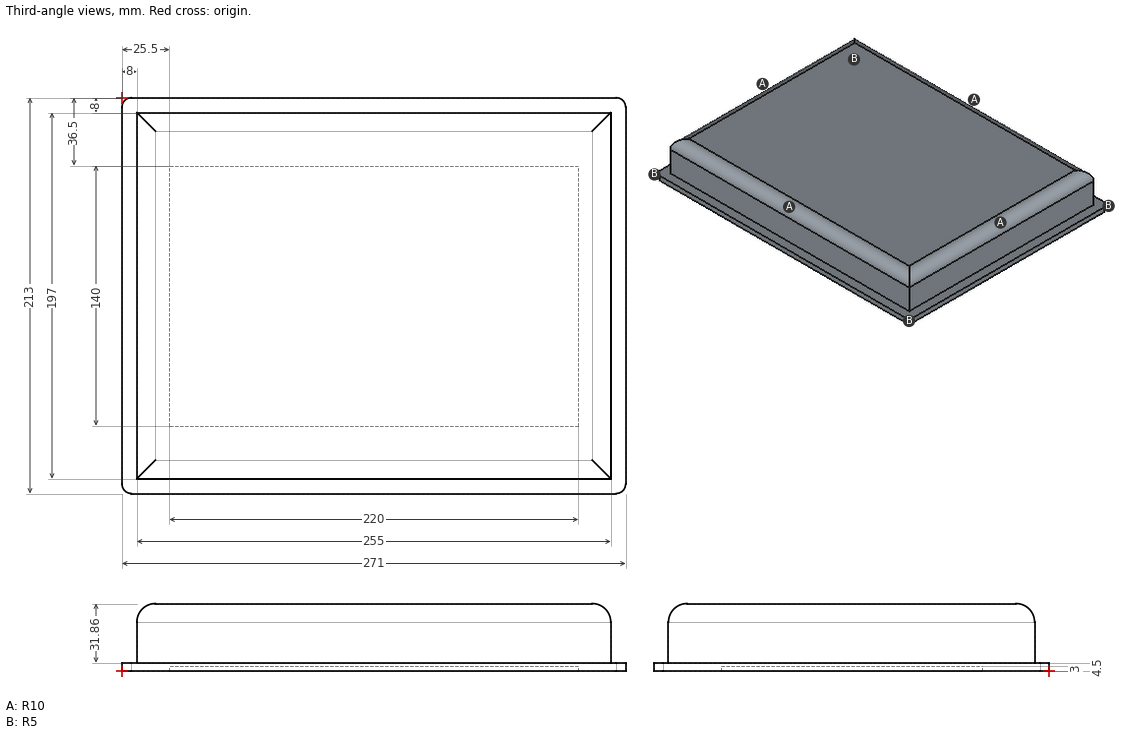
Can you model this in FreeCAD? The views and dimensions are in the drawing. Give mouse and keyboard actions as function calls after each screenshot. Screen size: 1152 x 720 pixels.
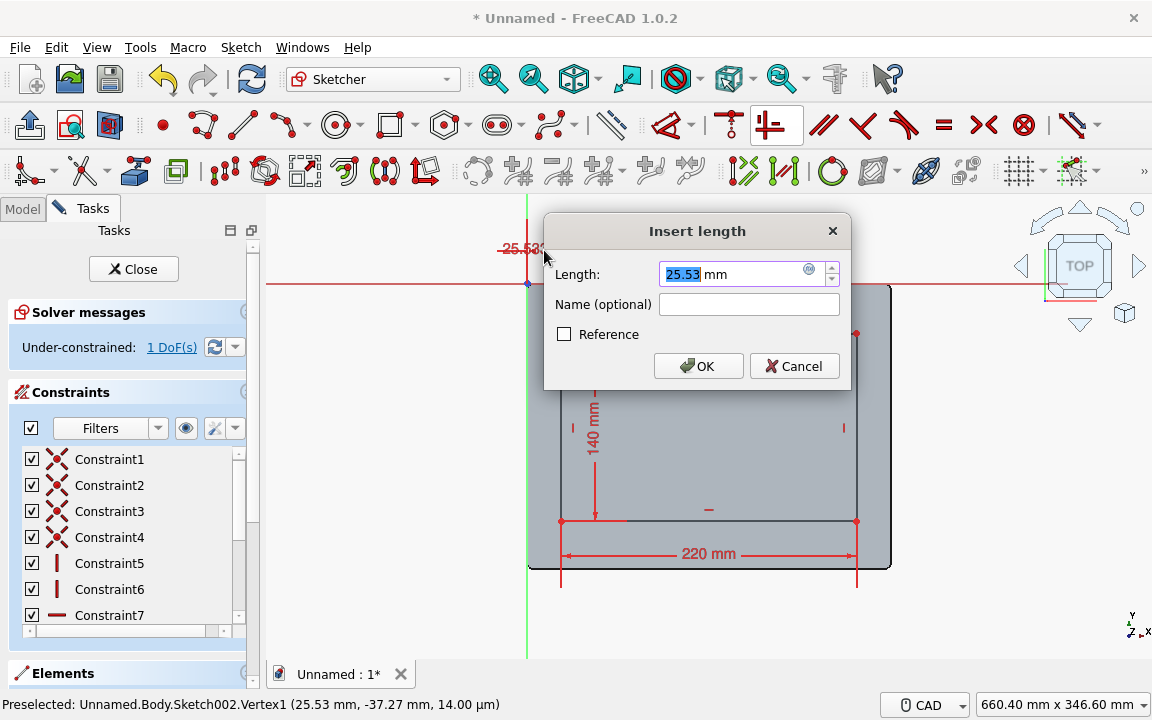
text(25.5)
key(Return)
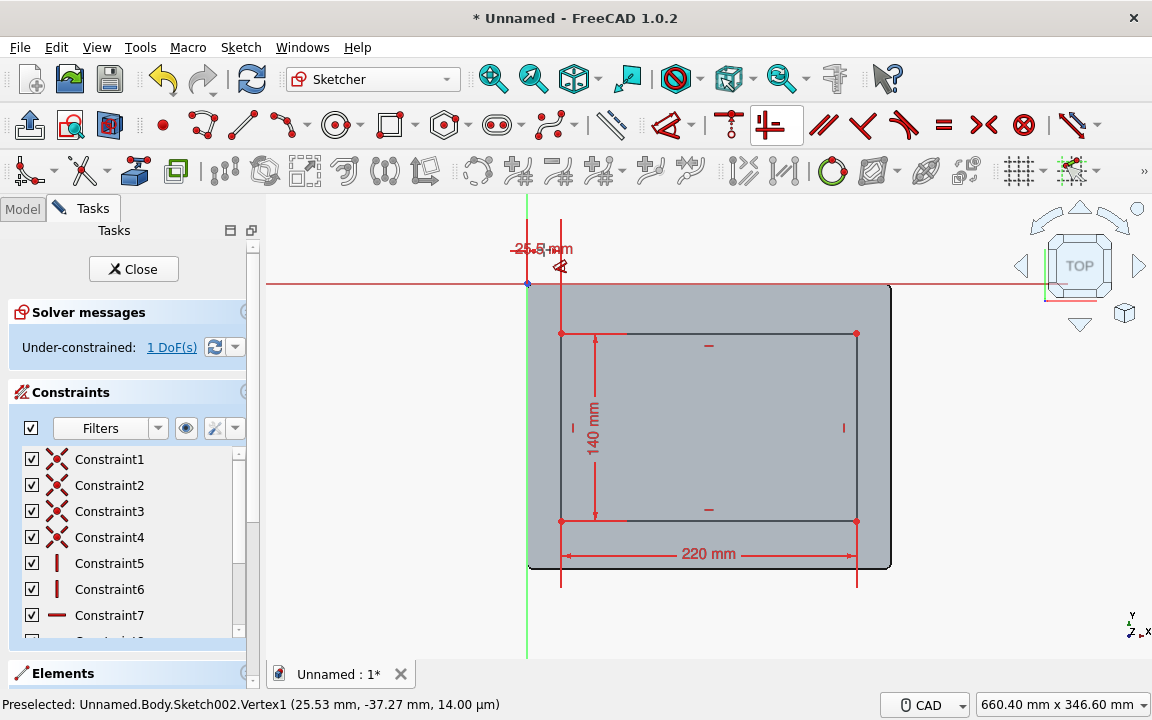
click(561, 334)
click(493, 309)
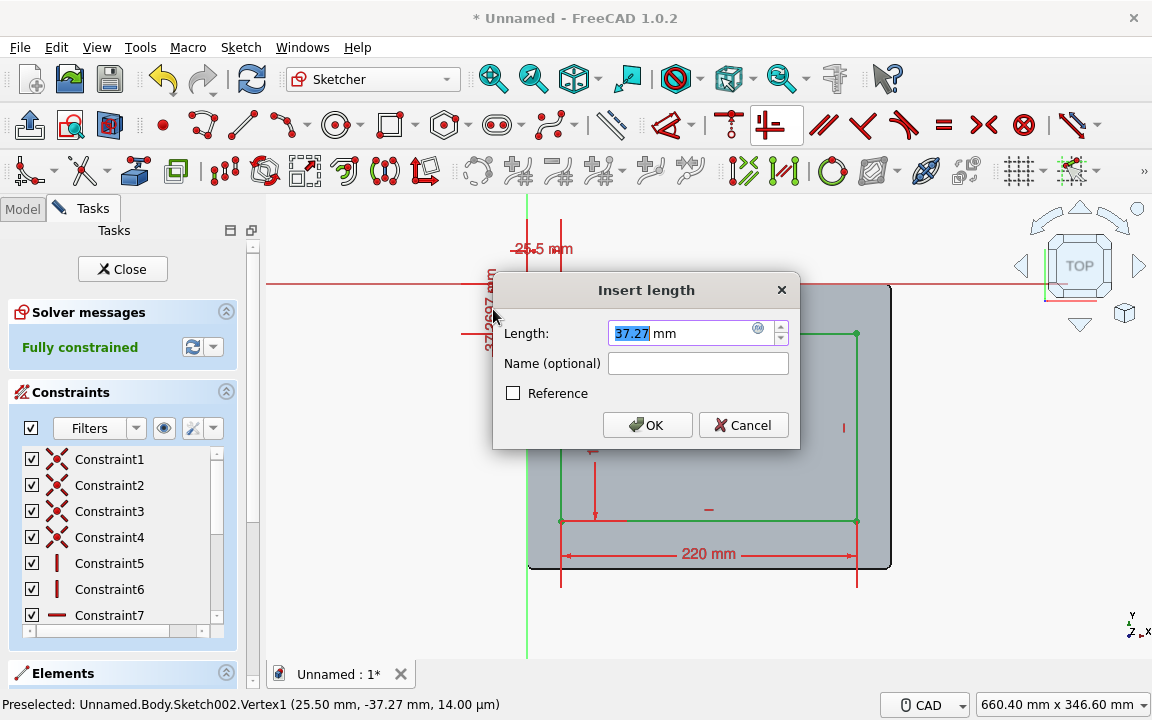
text(36.5)
key(Return)
key(Escape)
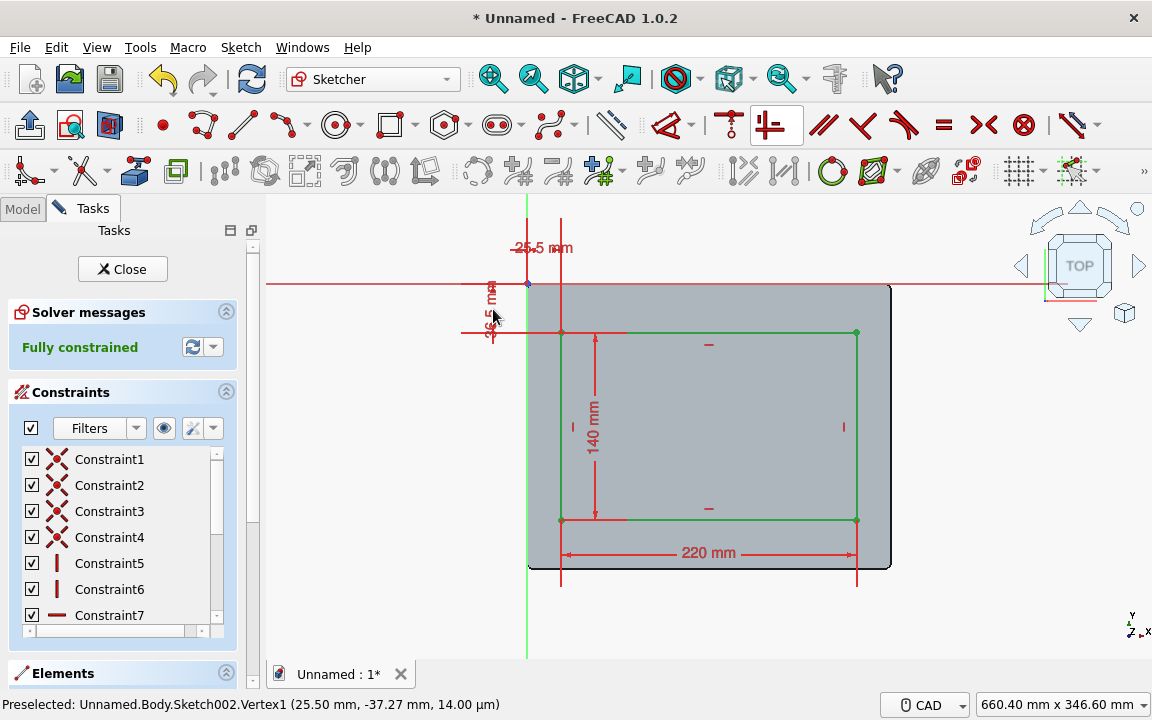
click(123, 269)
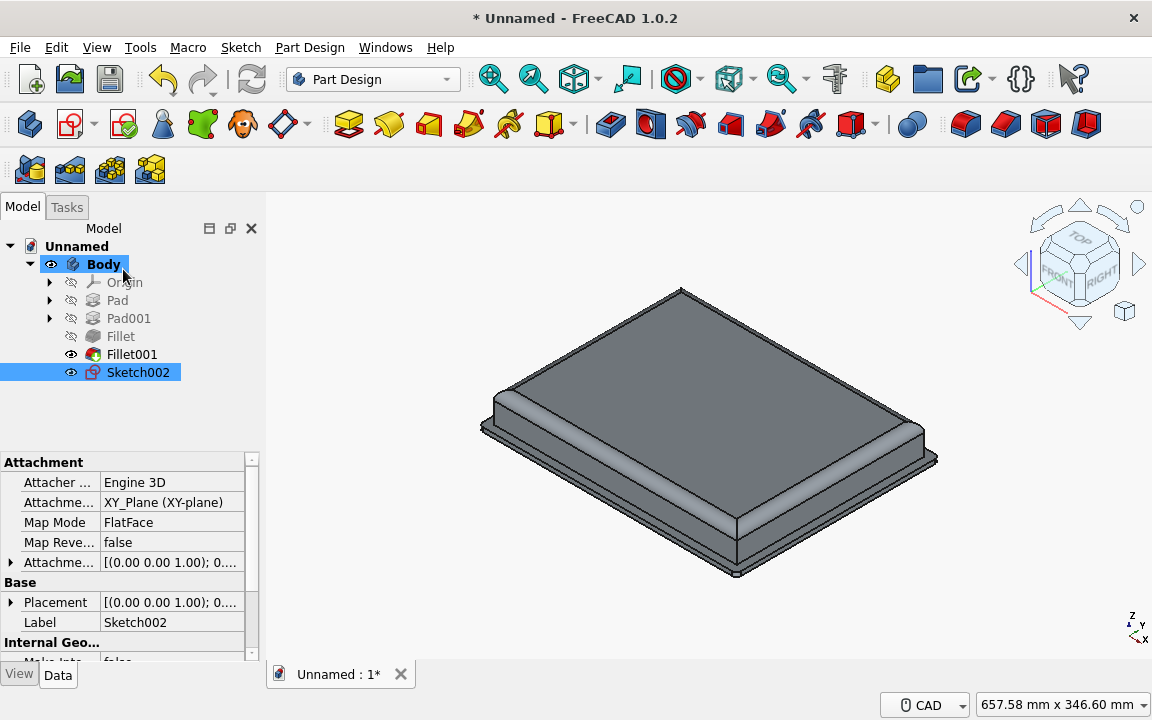
click(612, 124)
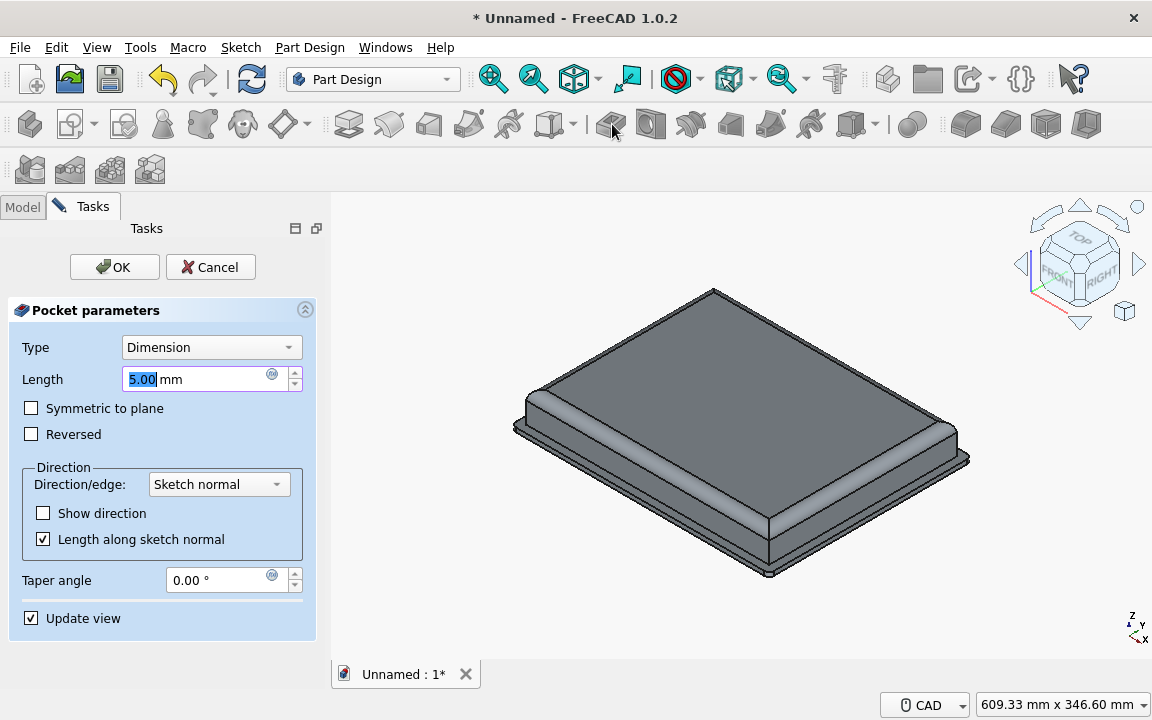
text(3)
key(Tab)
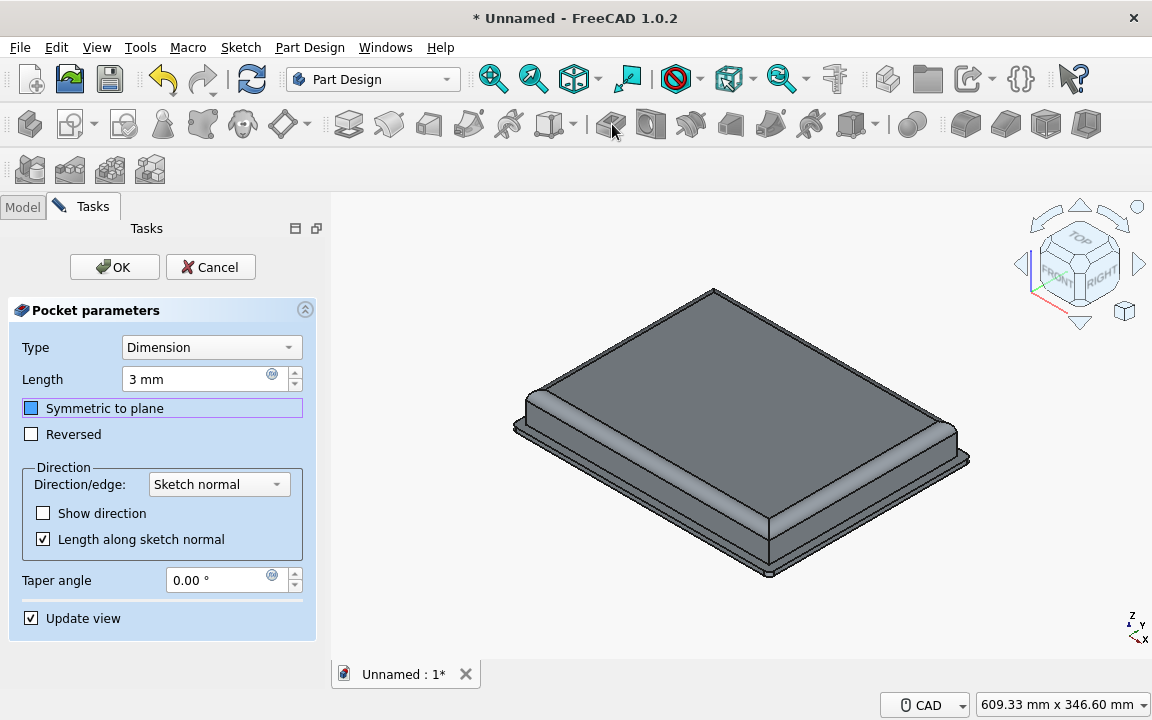
click(30, 434)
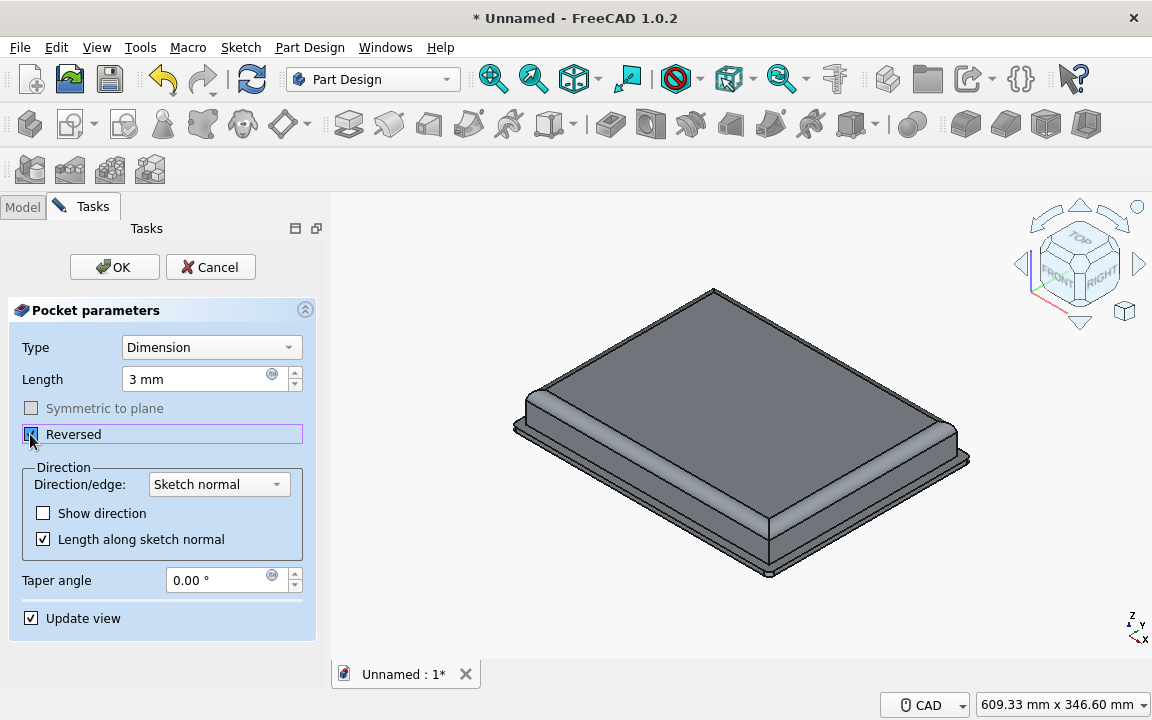
click(115, 267)